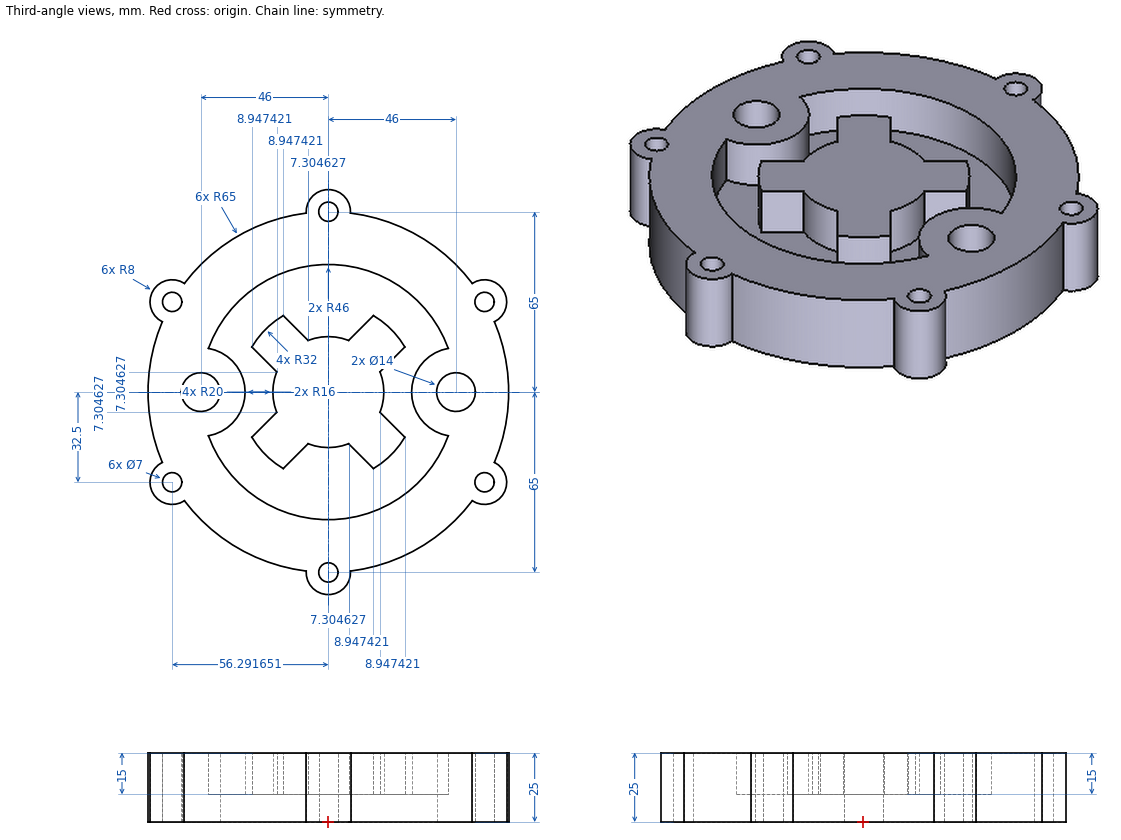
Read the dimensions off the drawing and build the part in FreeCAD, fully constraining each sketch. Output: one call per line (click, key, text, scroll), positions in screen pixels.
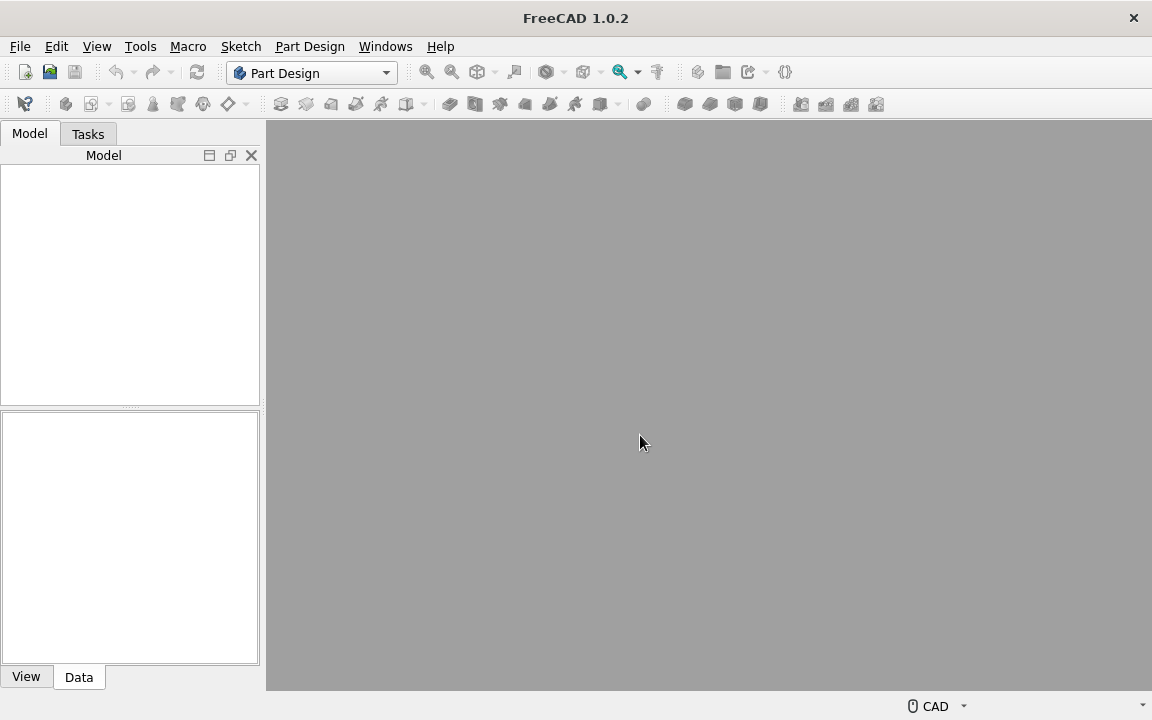
click(25, 72)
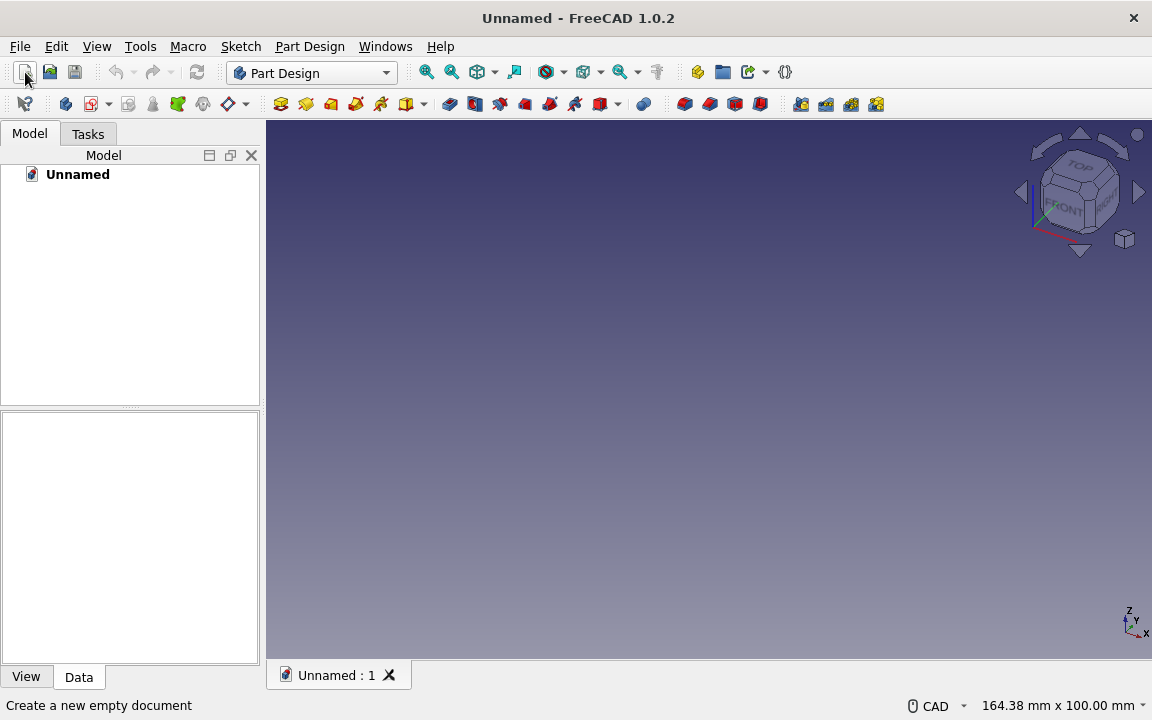
click(90, 104)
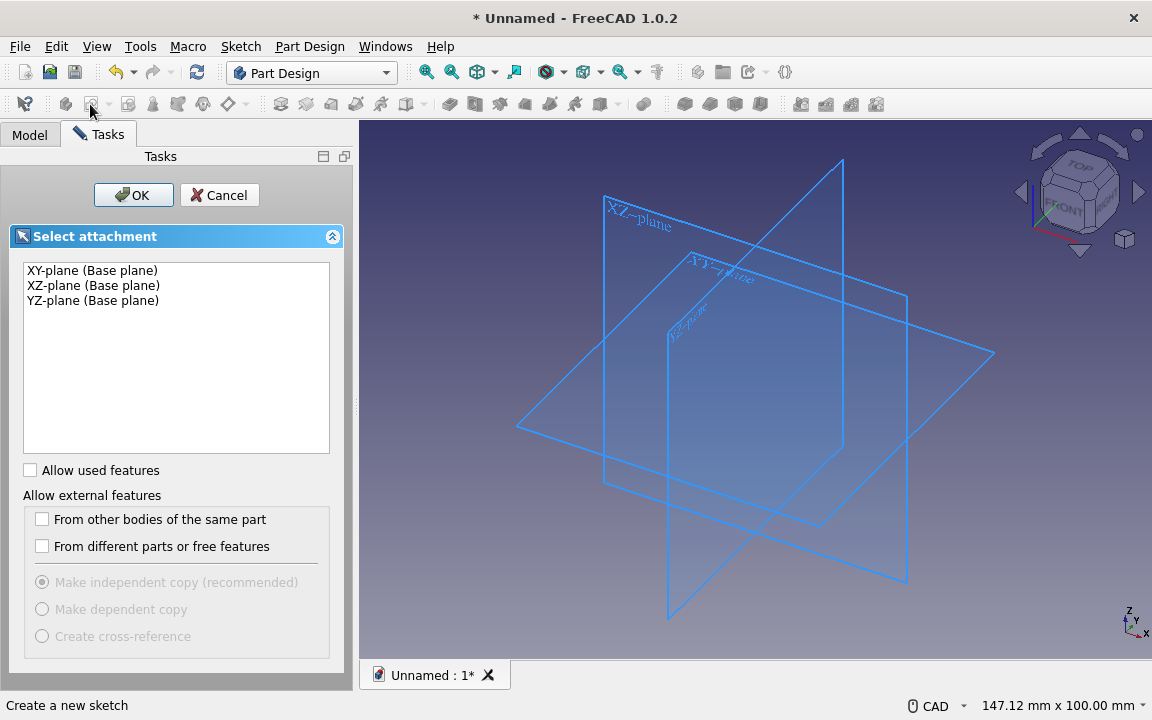
click(84, 270)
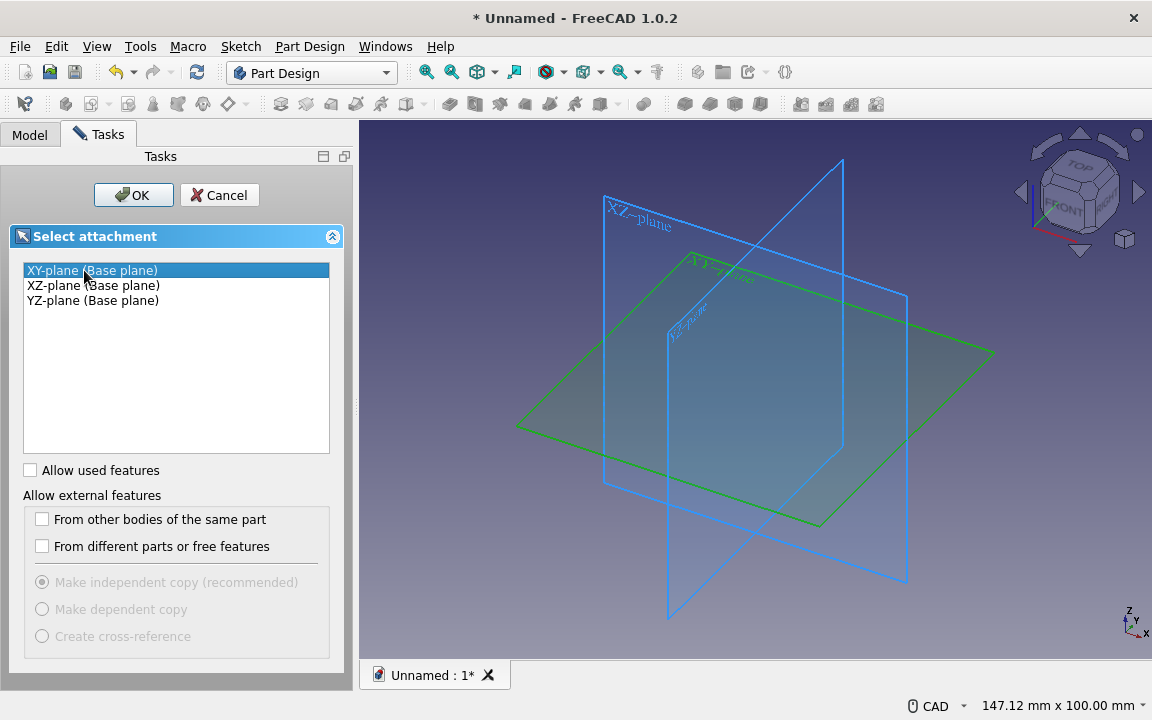
click(134, 195)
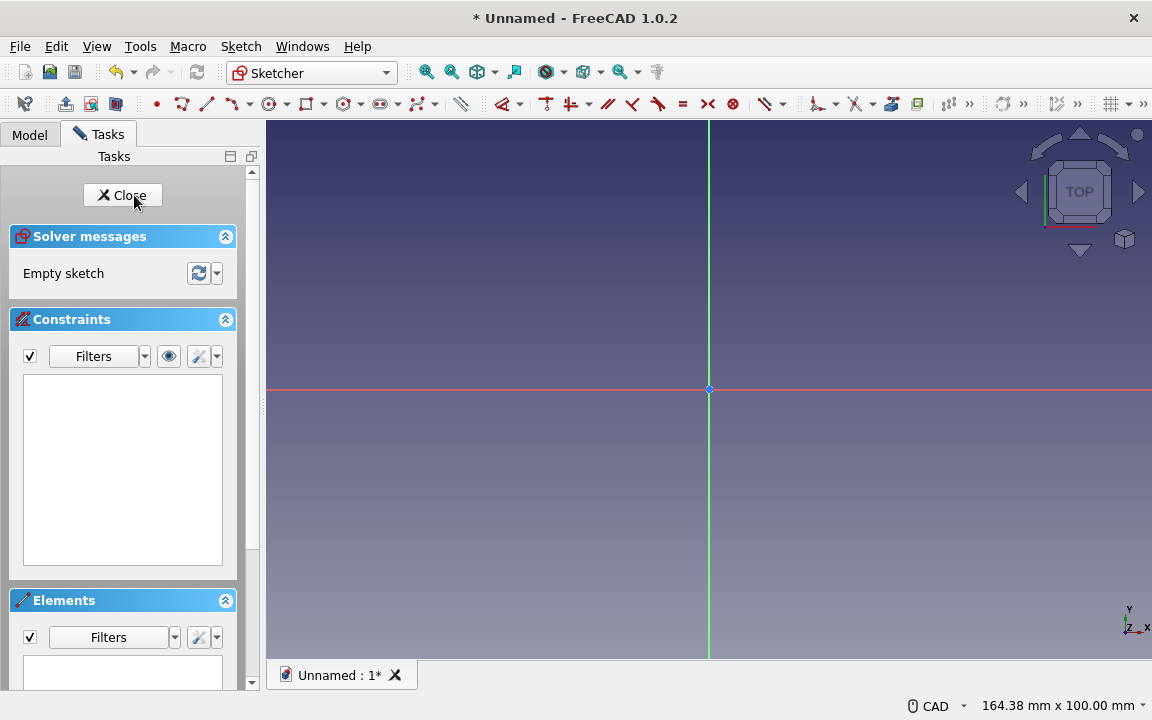
scroll(585, 390, down, 4)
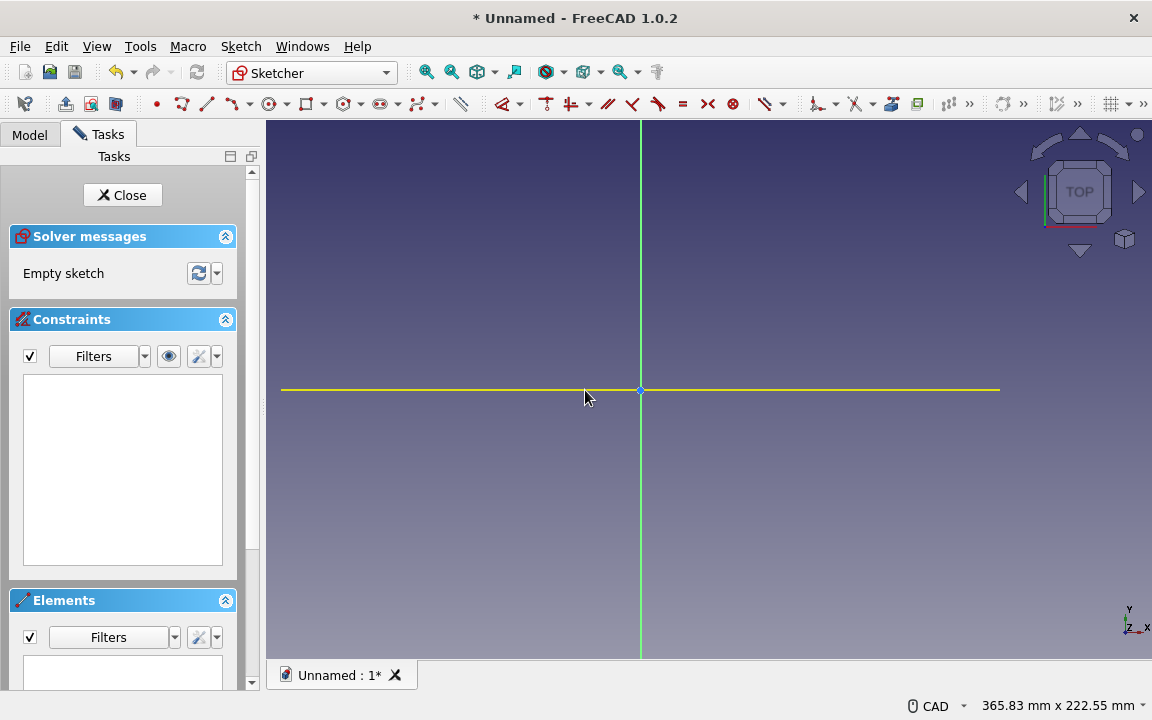
click(232, 104)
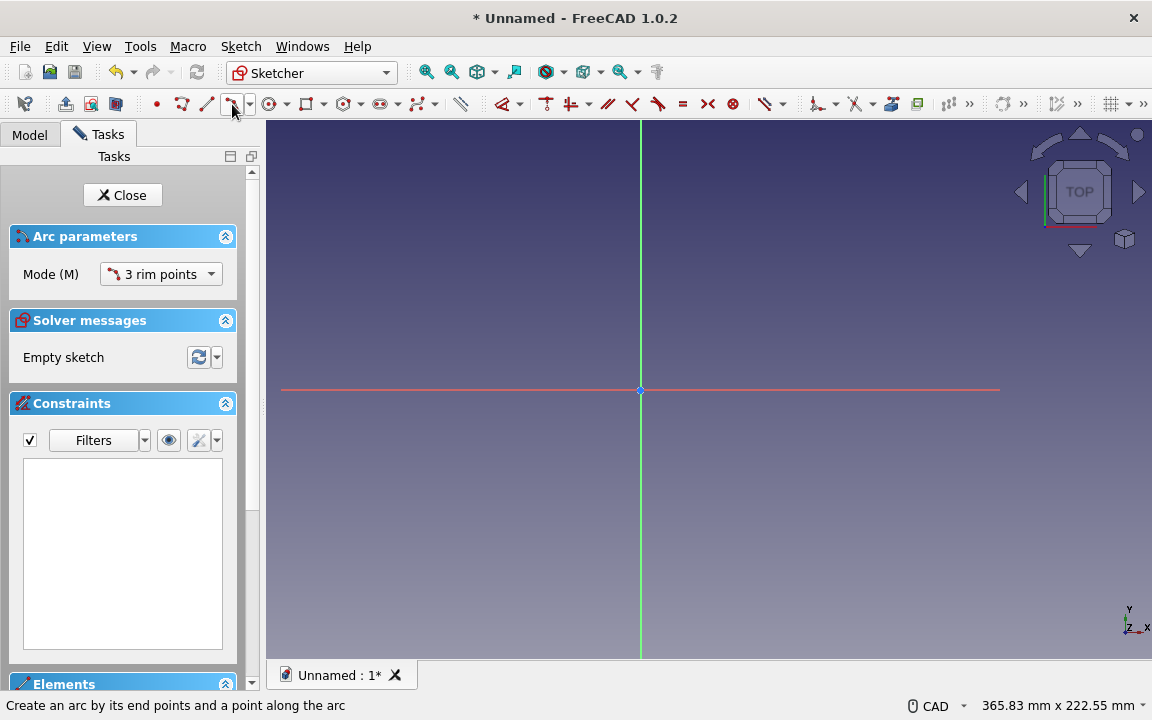
click(496, 329)
click(496, 451)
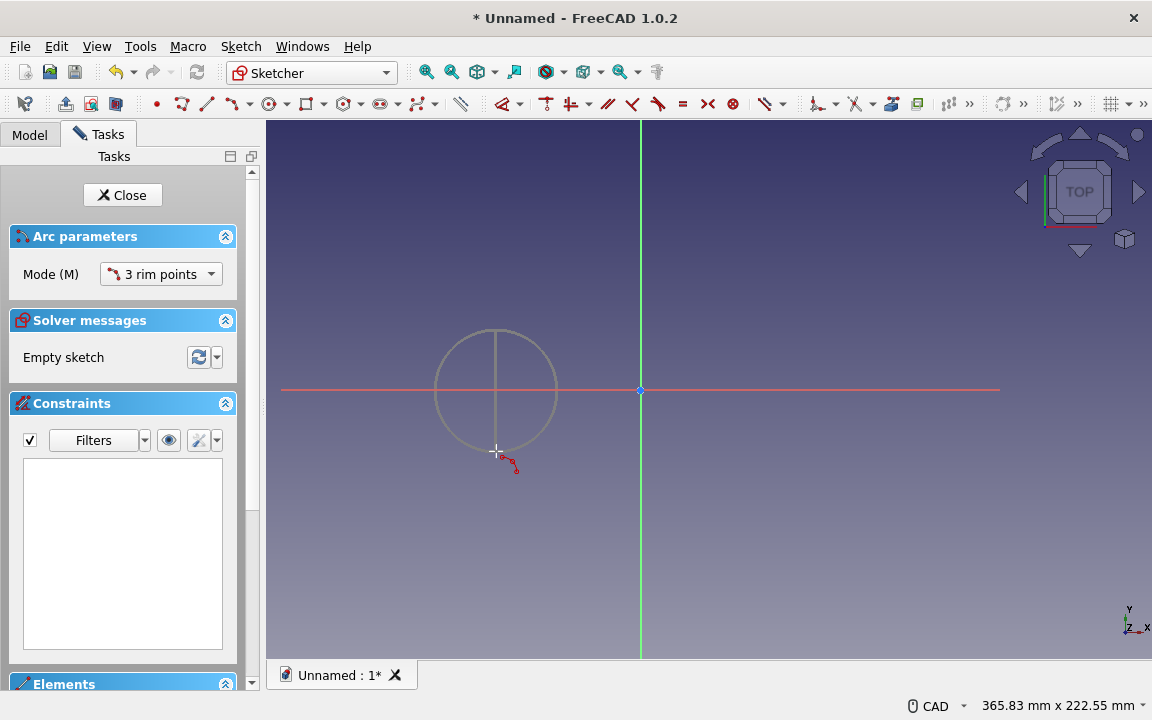
scroll(484, 377, up, 2)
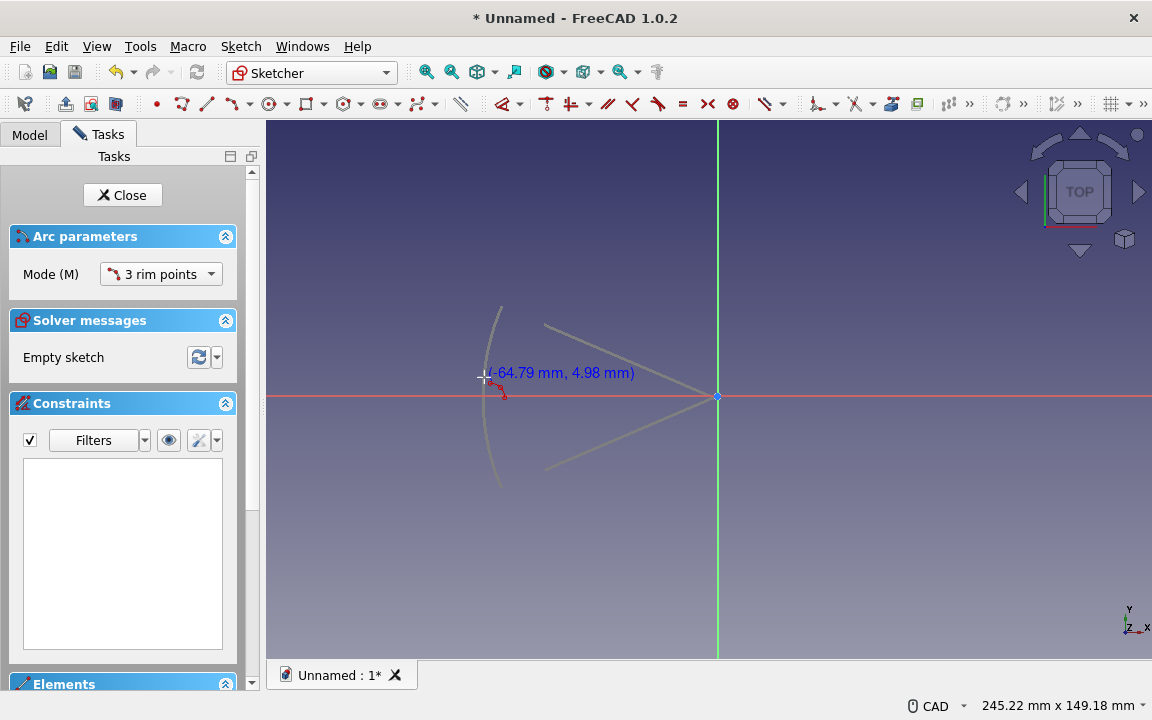
click(484, 377)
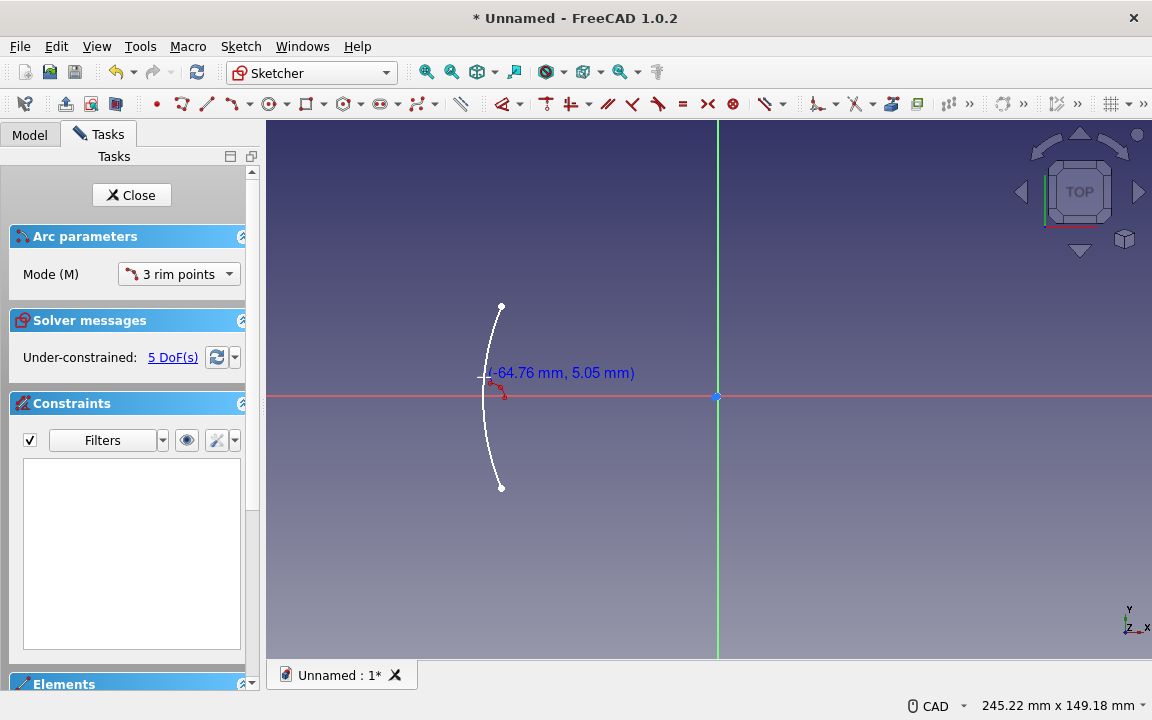
click(502, 489)
click(531, 538)
click(490, 528)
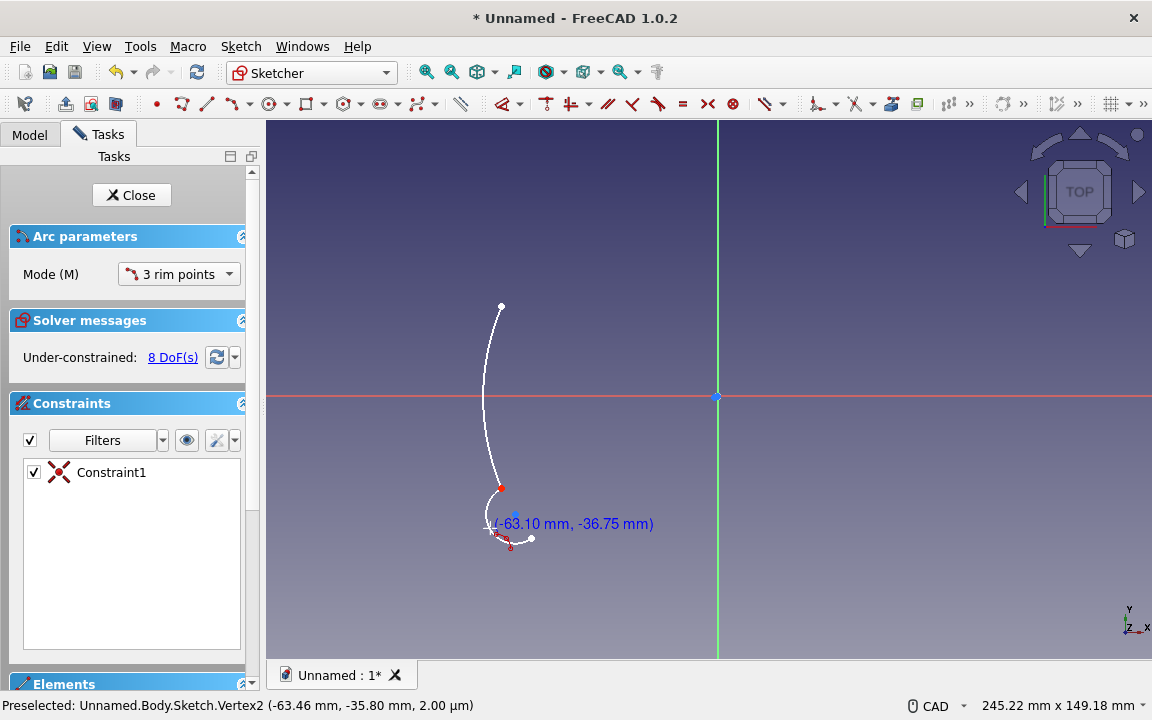
click(531, 539)
click(689, 629)
click(601, 600)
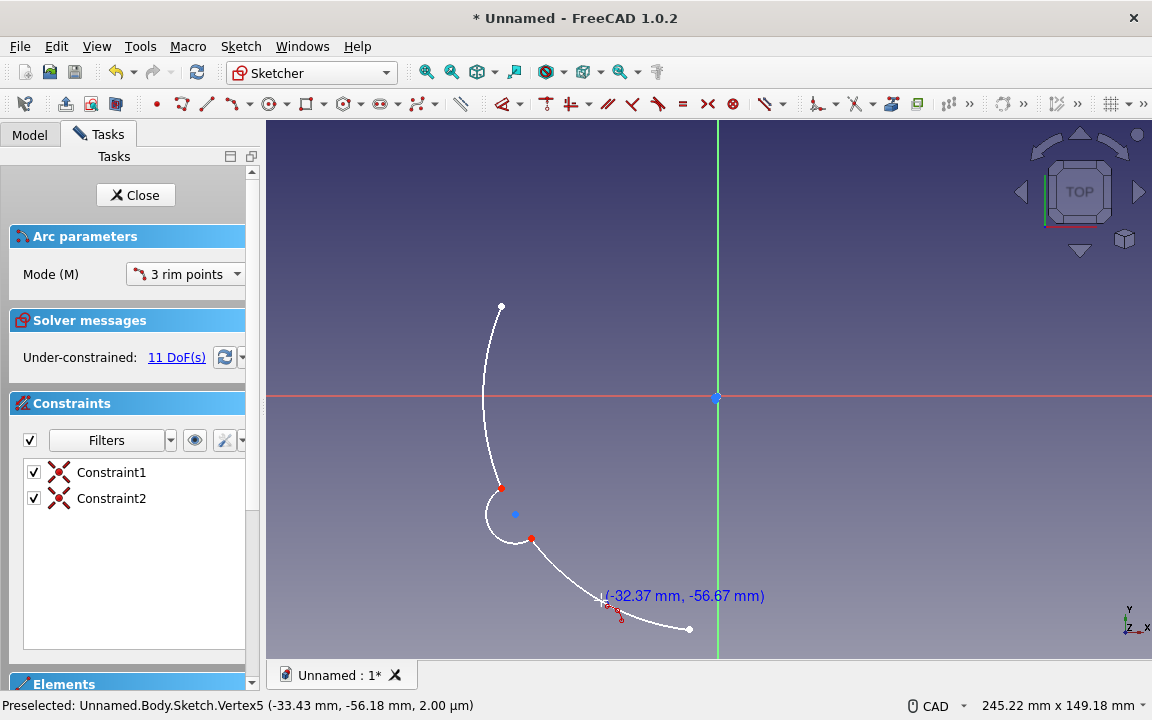
click(689, 630)
click(747, 629)